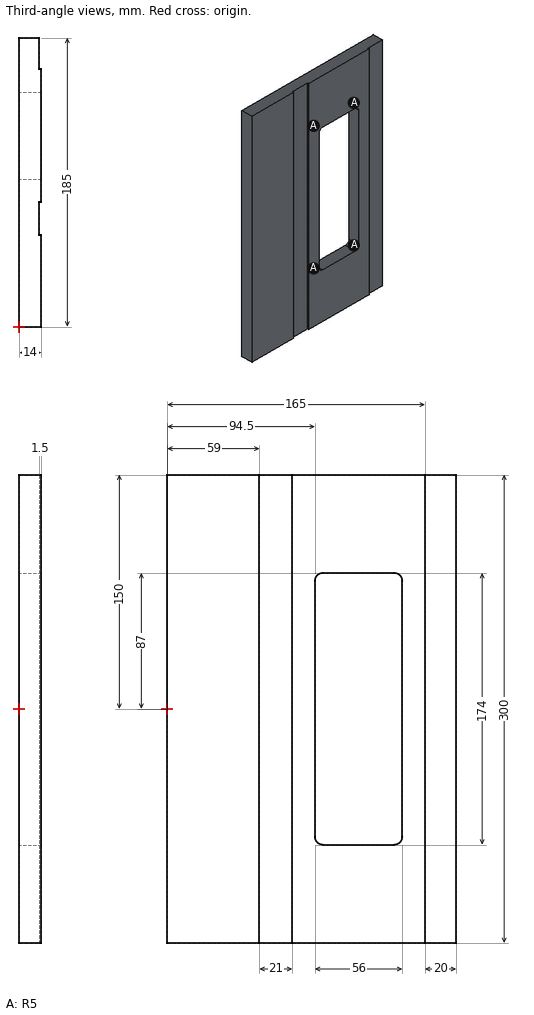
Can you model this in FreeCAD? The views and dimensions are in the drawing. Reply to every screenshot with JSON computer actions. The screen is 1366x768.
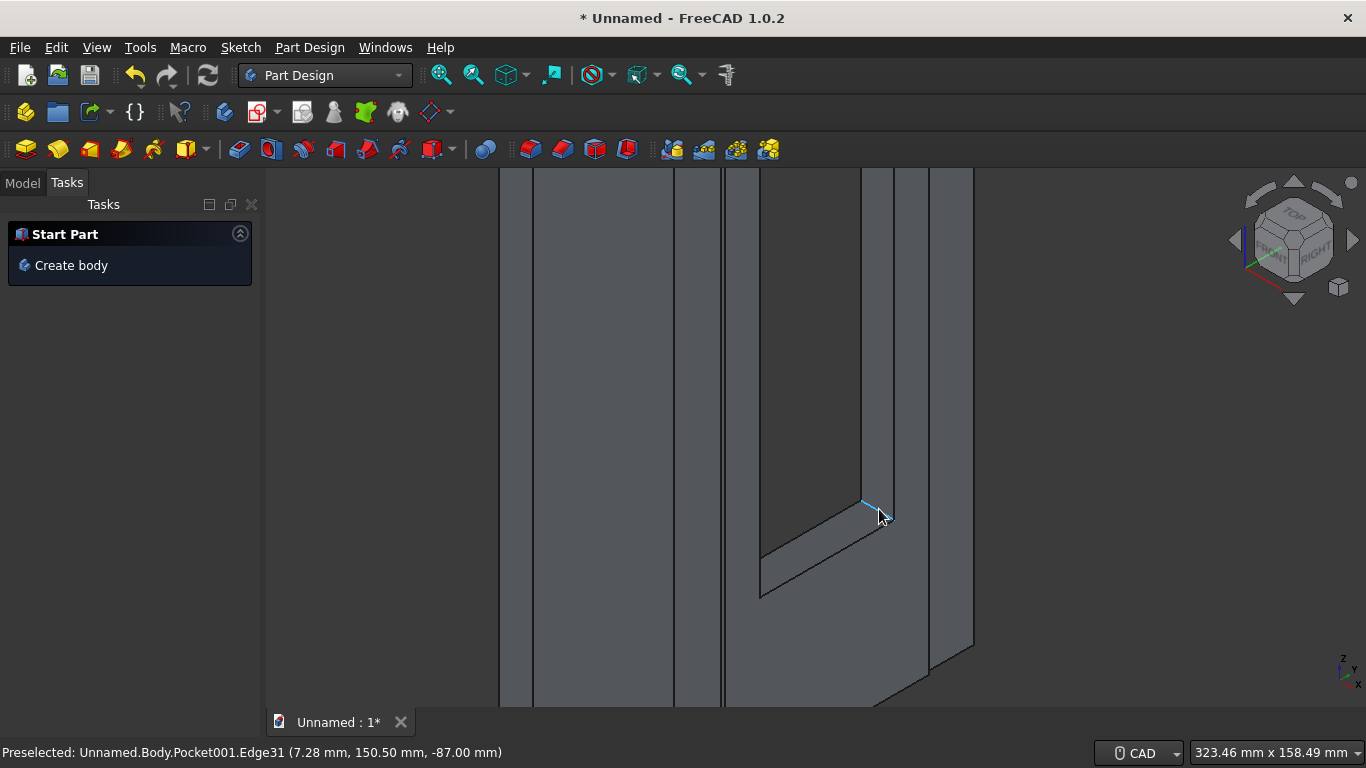
{"action": "left_click", "coordinate": [442, 76]}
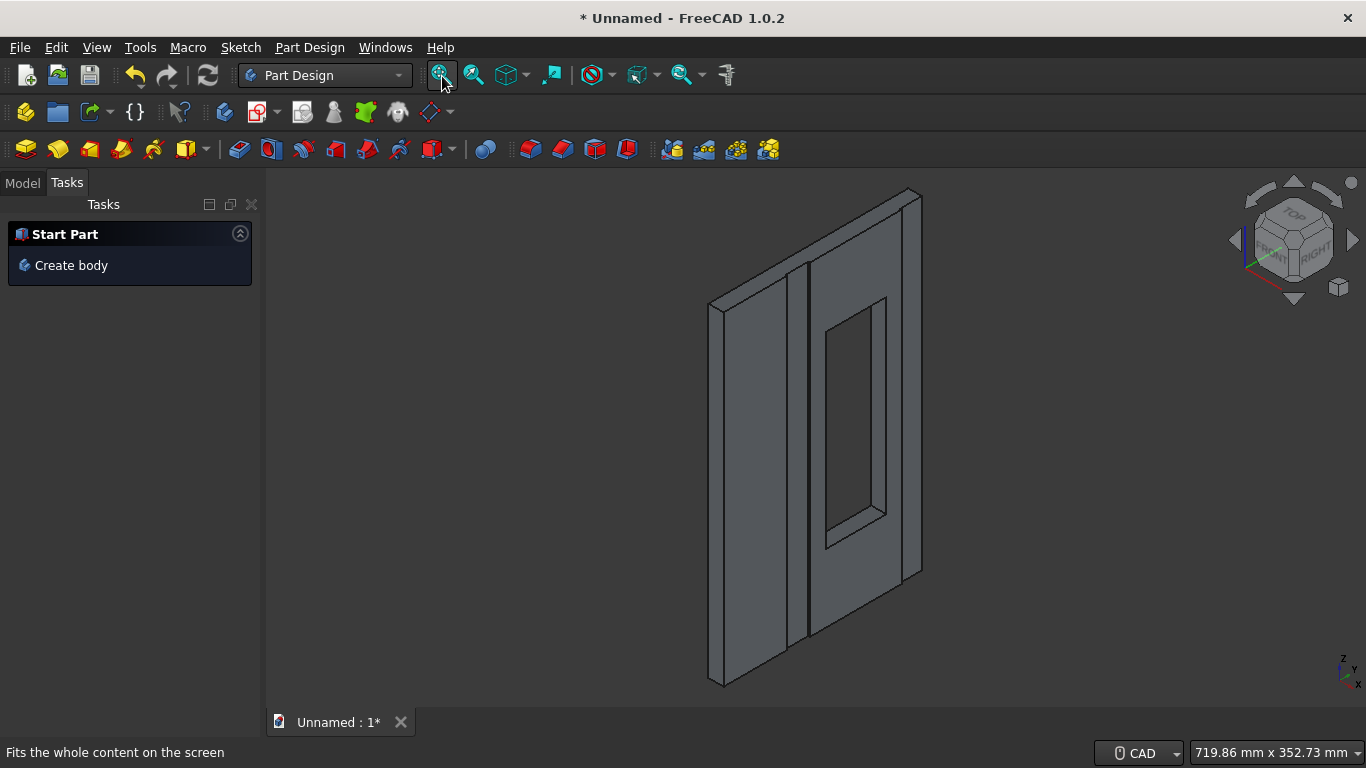
{"action": "key", "text": "2"}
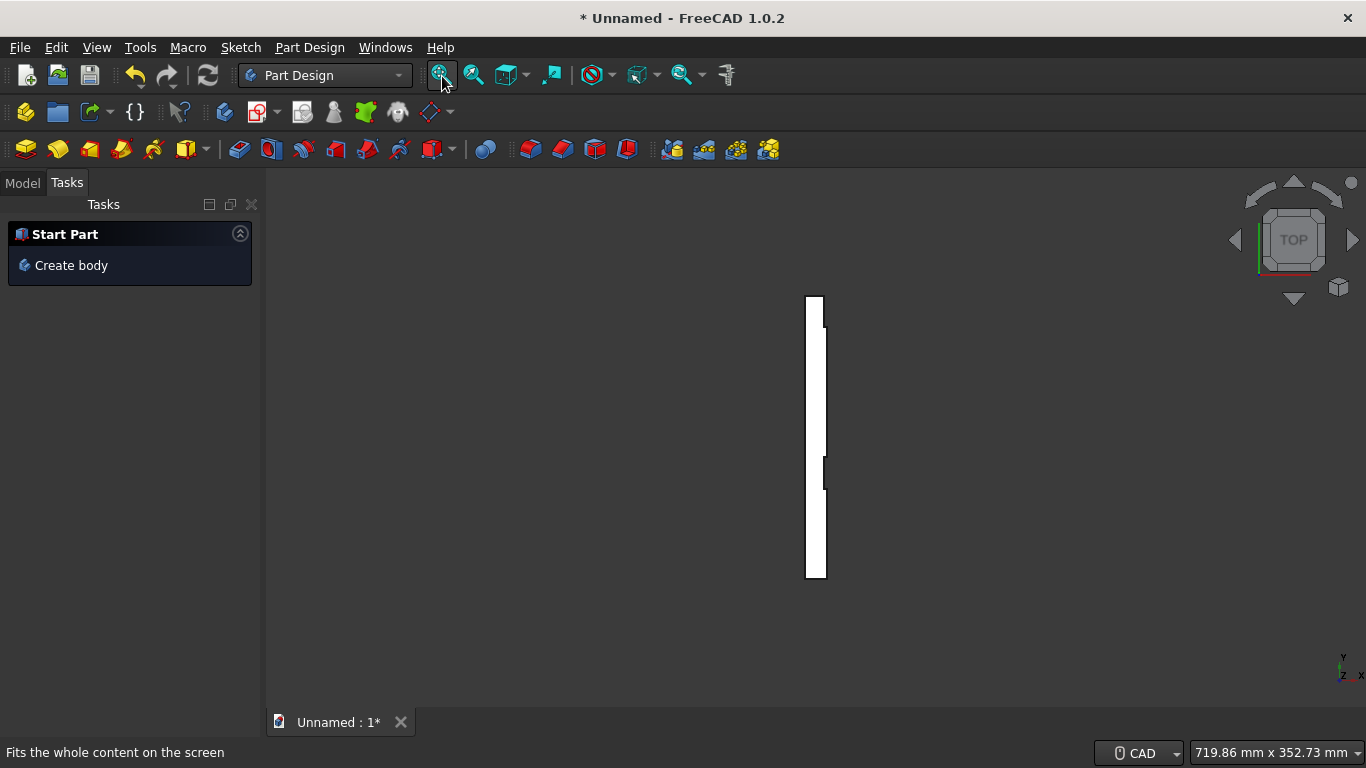
{"action": "scroll", "coordinate": [816, 348], "scroll_direction": "up", "scroll_amount": 4}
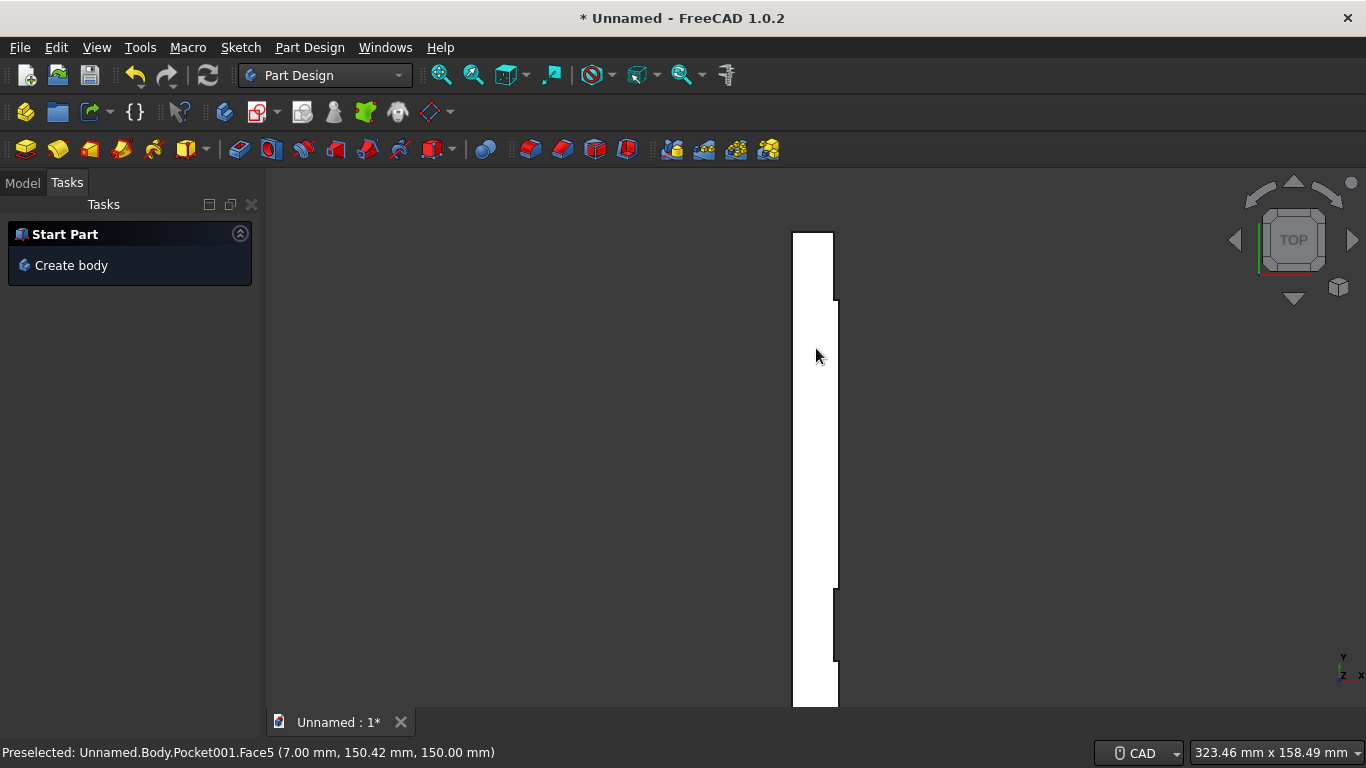
{"action": "left_click", "coordinate": [442, 76]}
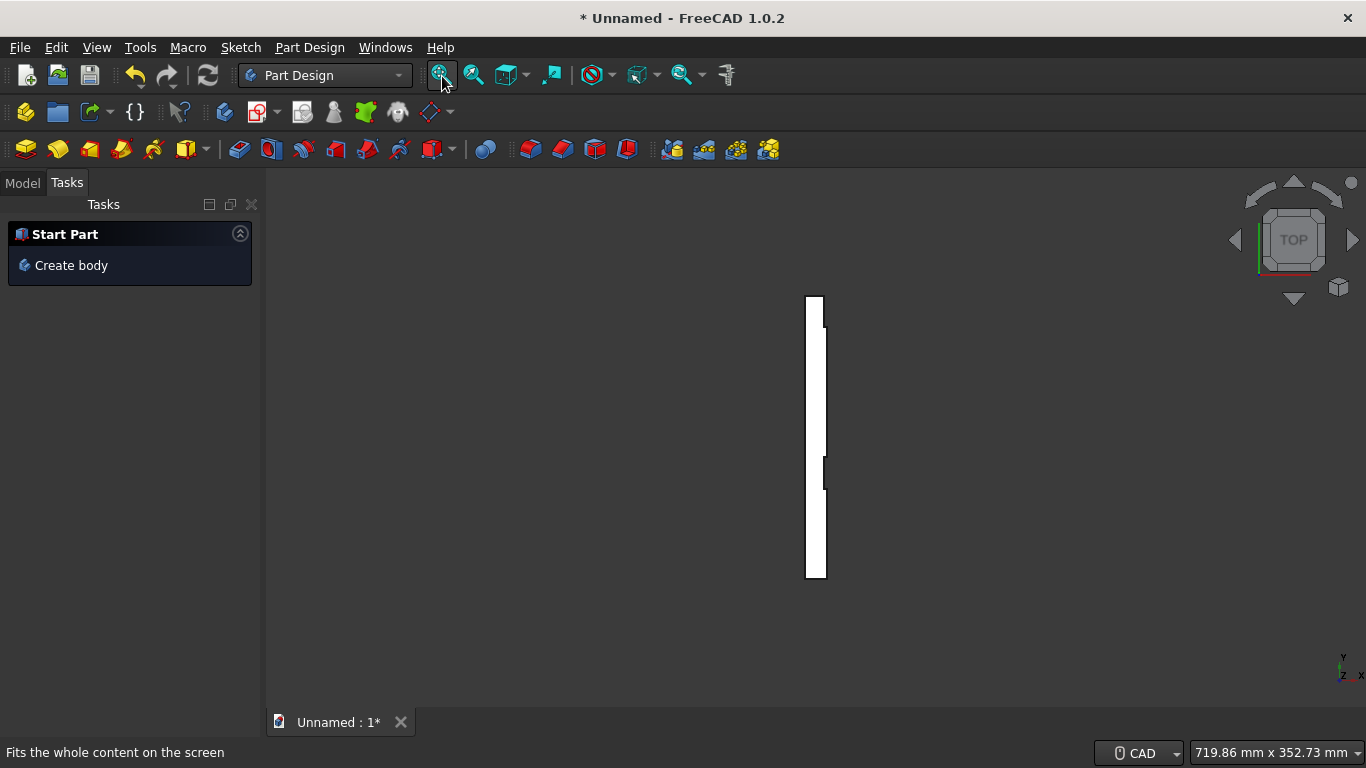
{"action": "key", "text": "1"}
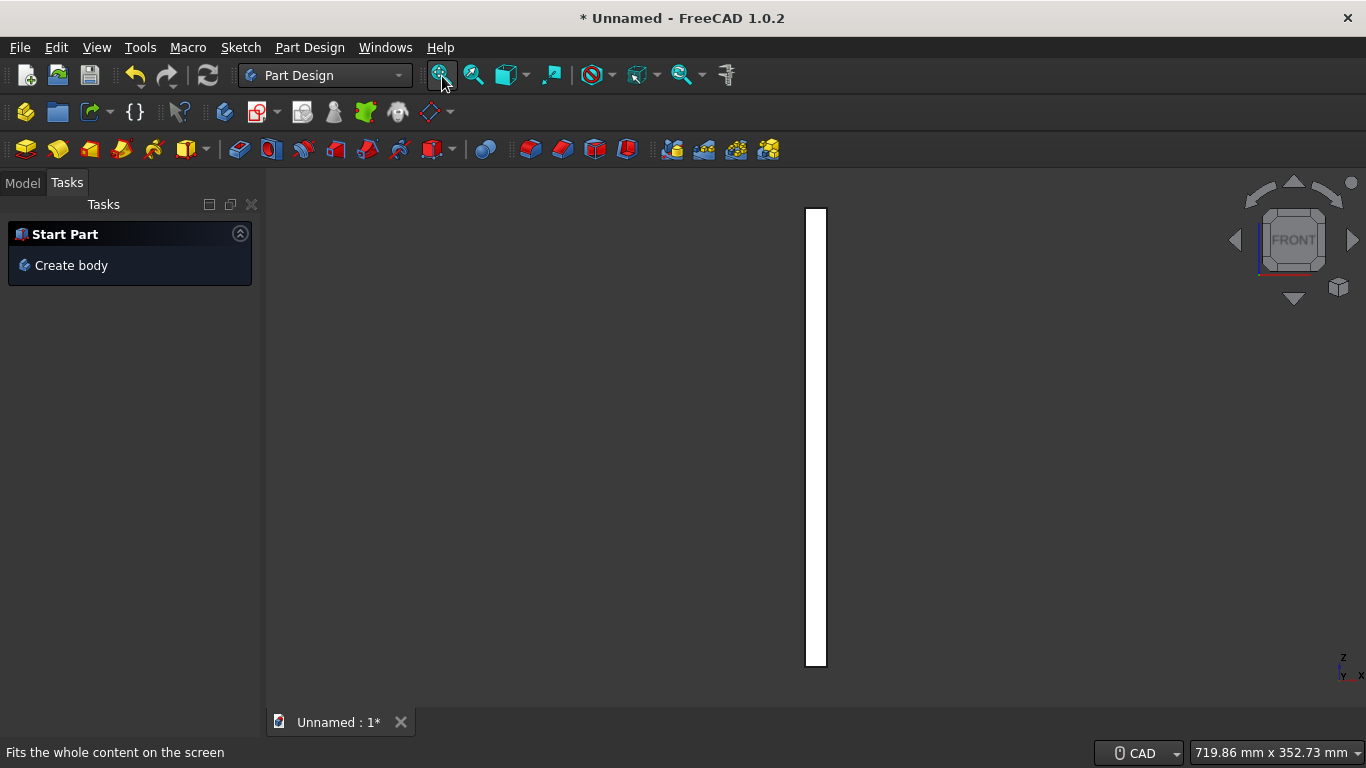
{"action": "scroll", "coordinate": [816, 569], "scroll_direction": "up", "scroll_amount": 4}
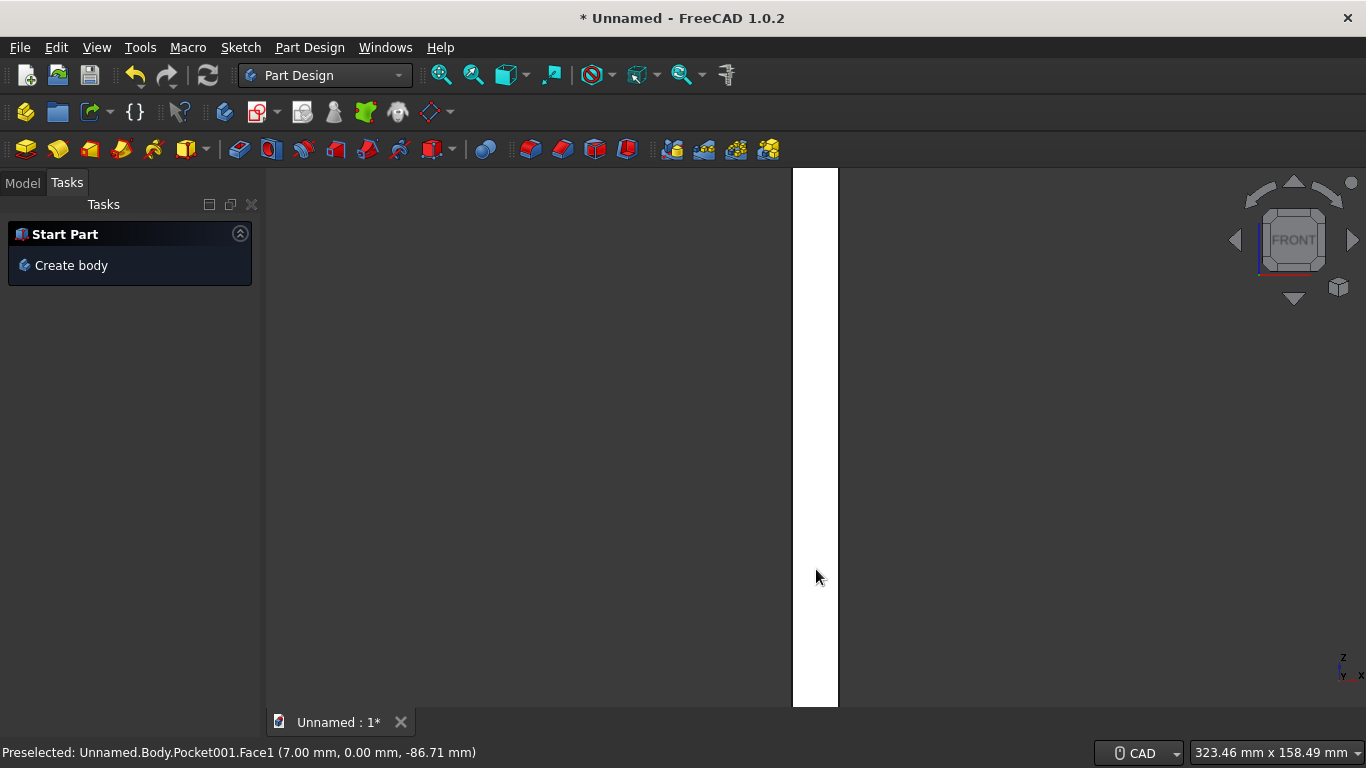
{"action": "key", "text": "v f"}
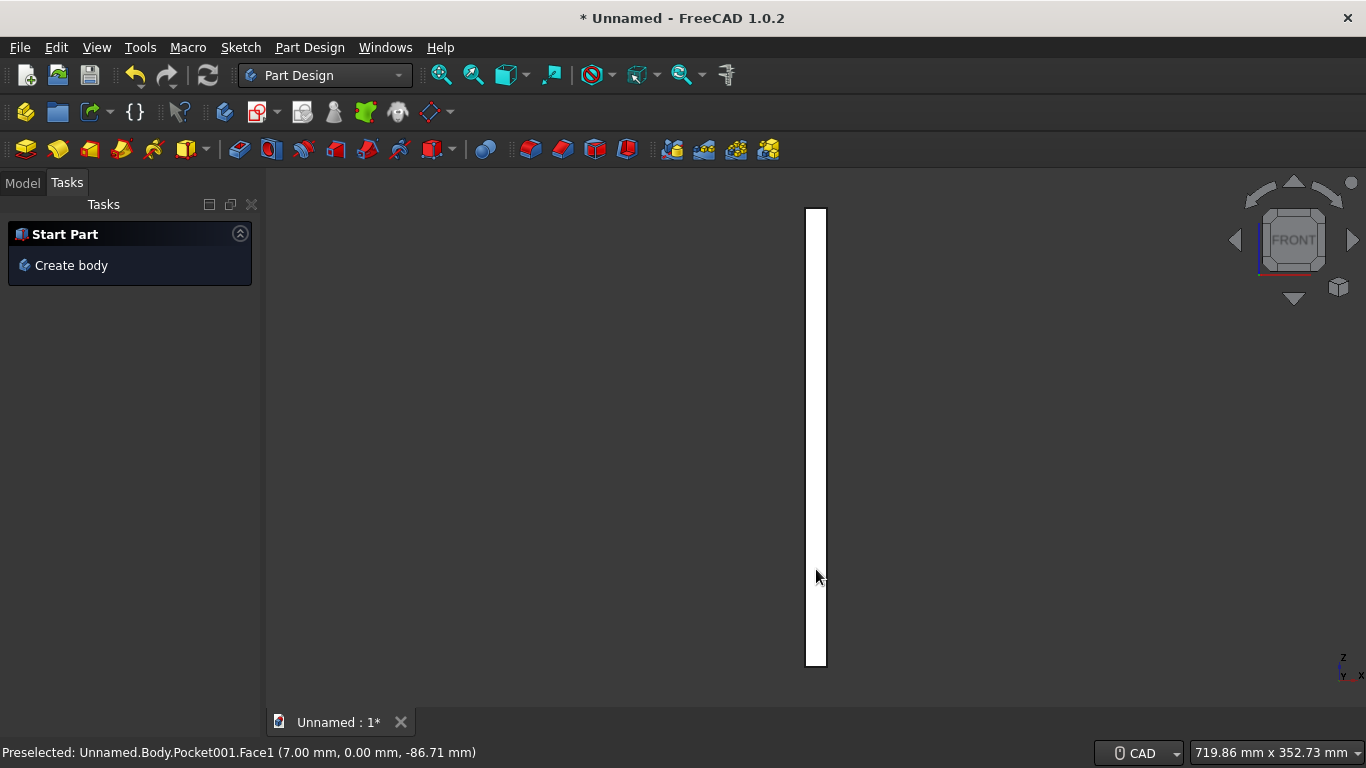
{"action": "key", "text": "3"}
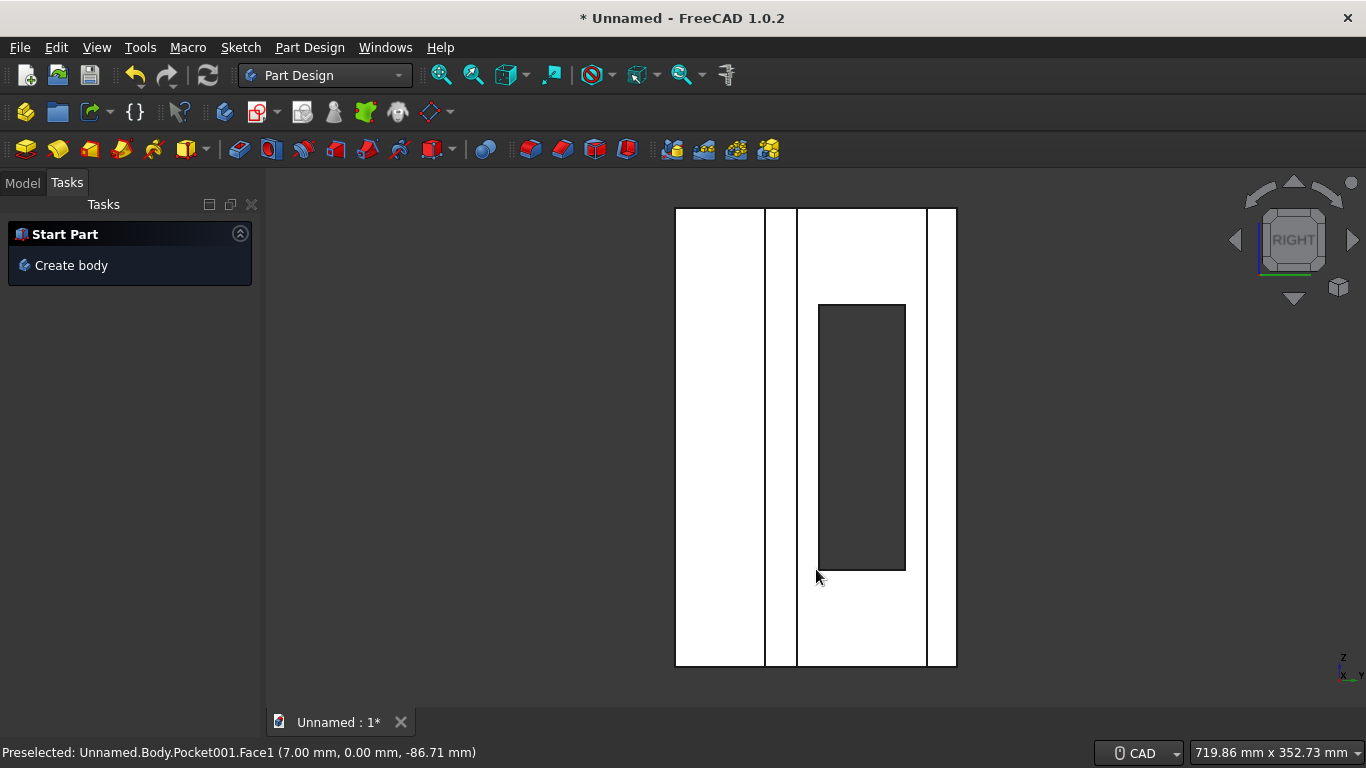
{"action": "scroll", "coordinate": [905, 569], "scroll_direction": "up", "scroll_amount": 4}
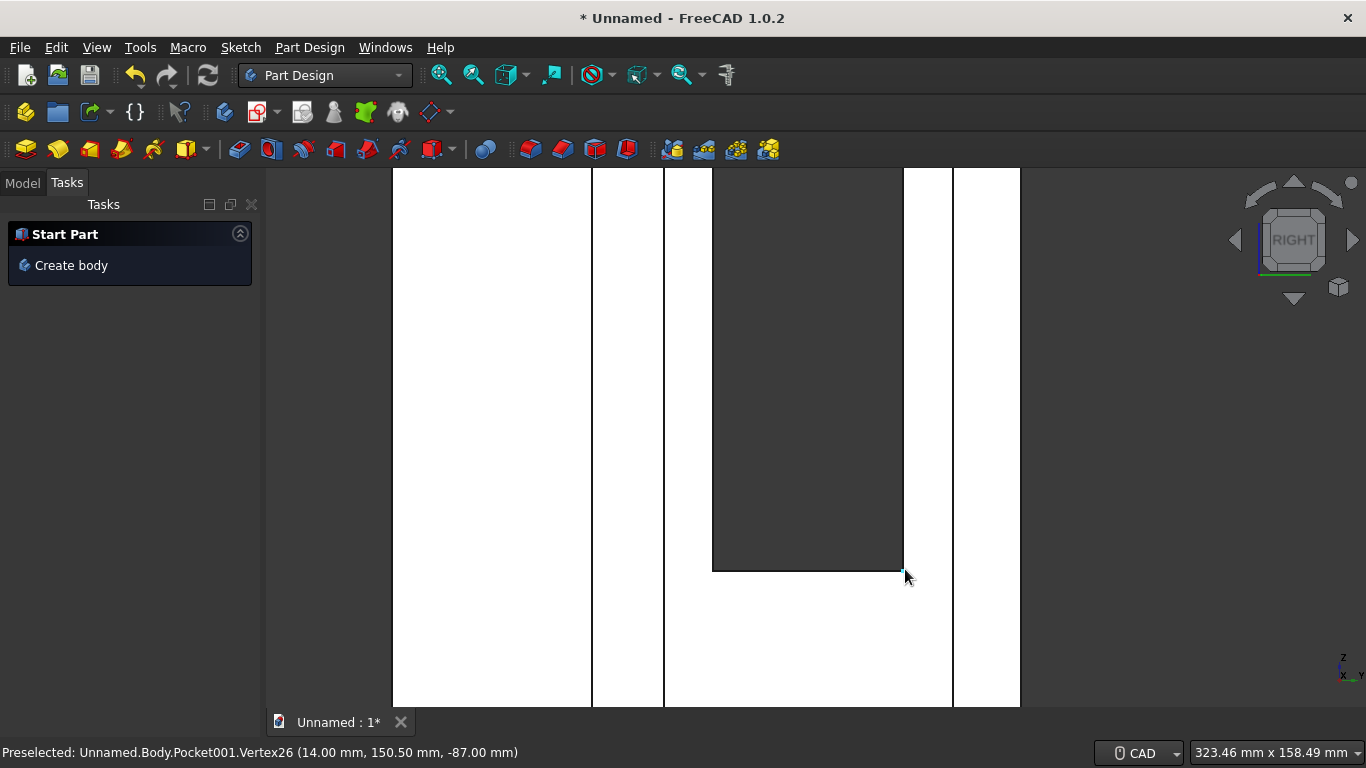
{"action": "key", "text": "v f"}